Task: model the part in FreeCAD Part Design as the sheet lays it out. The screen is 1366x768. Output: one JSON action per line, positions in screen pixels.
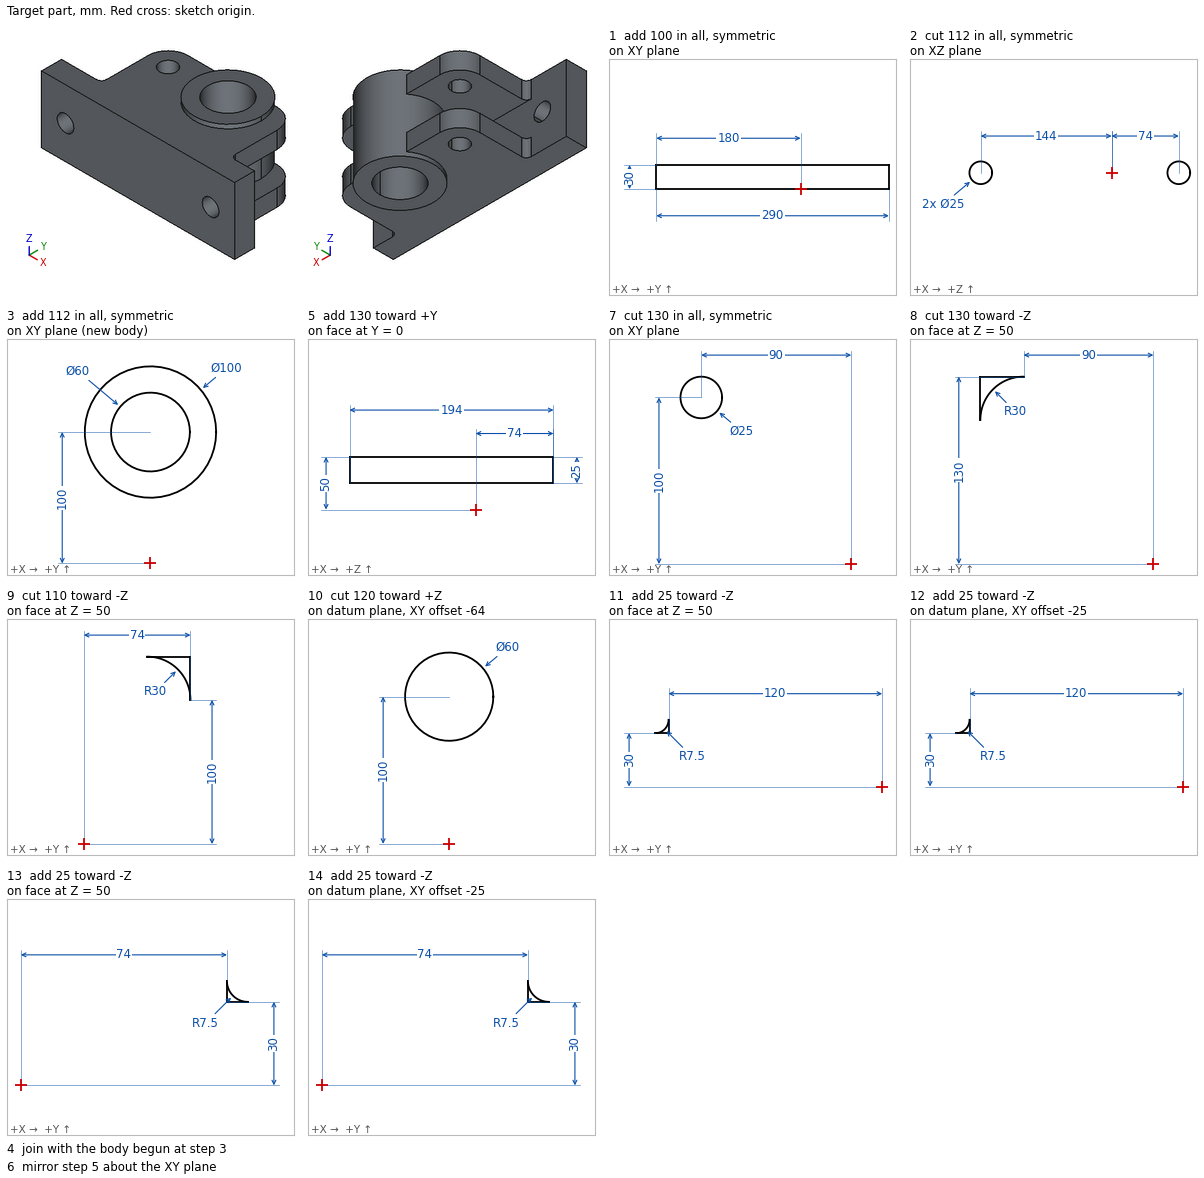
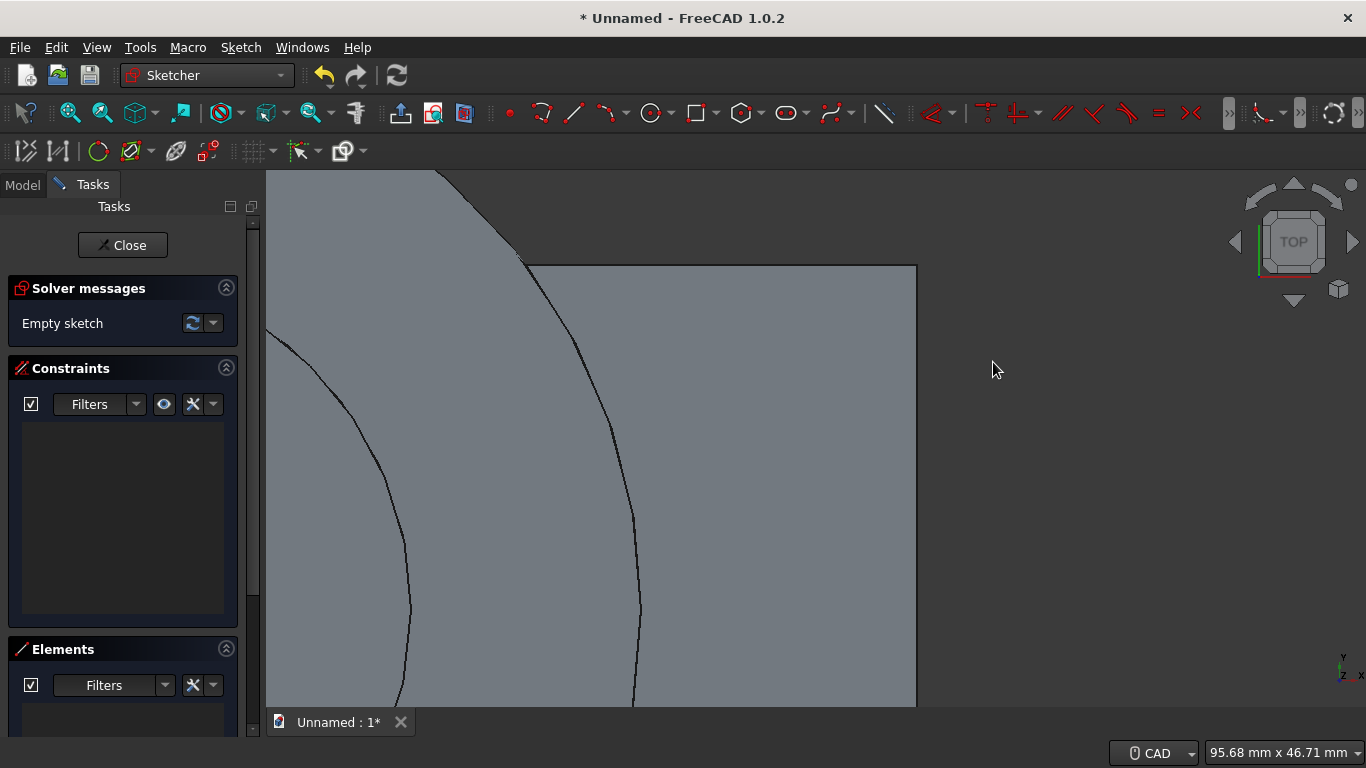
{"action": "left_click", "coordinate": [542, 114]}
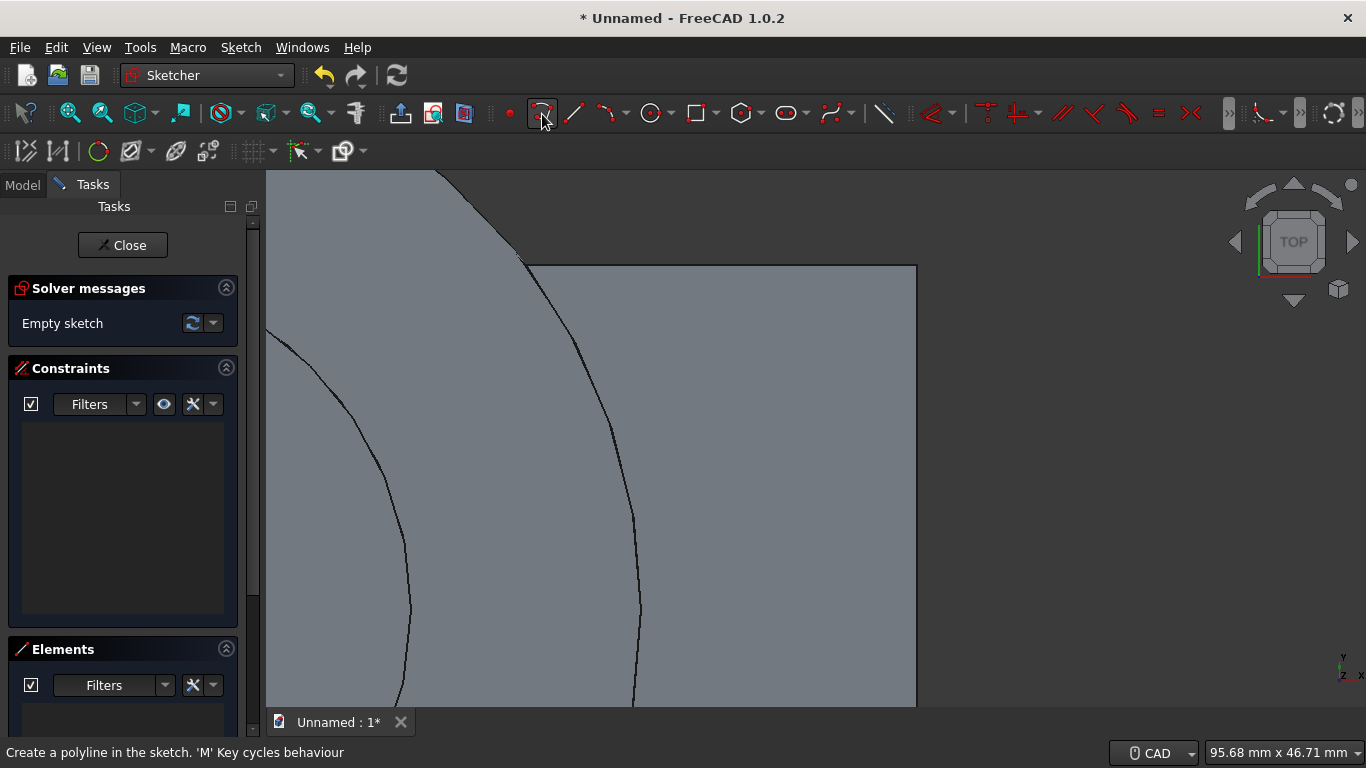
{"action": "left_click", "coordinate": [917, 610]}
{"action": "left_click", "coordinate": [917, 265]}
{"action": "left_click", "coordinate": [572, 265]}
{"action": "right_click", "coordinate": [572, 265]}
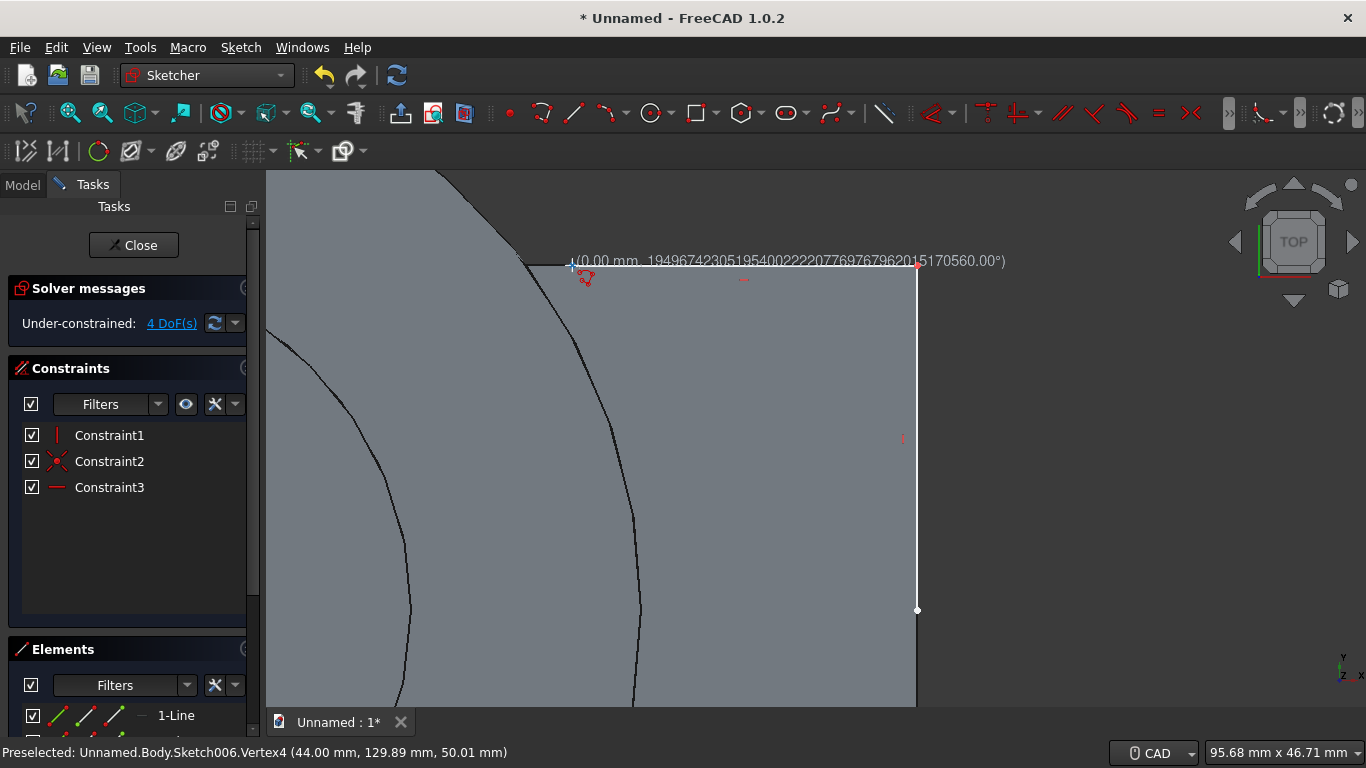
{"action": "left_click", "coordinate": [606, 114]}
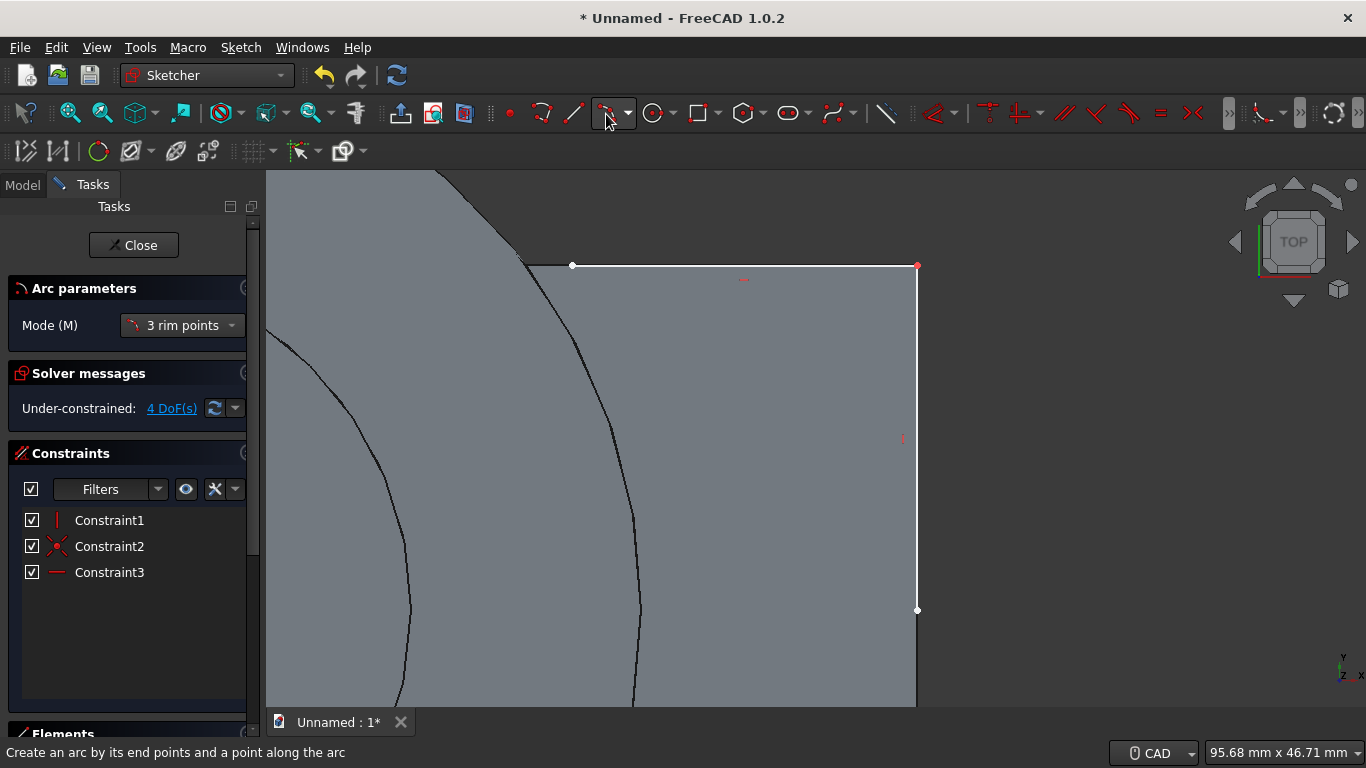
{"action": "left_click", "coordinate": [572, 266]}
{"action": "left_click", "coordinate": [917, 611]}
{"action": "left_click", "coordinate": [816, 366]}
{"action": "key", "text": "Escape"}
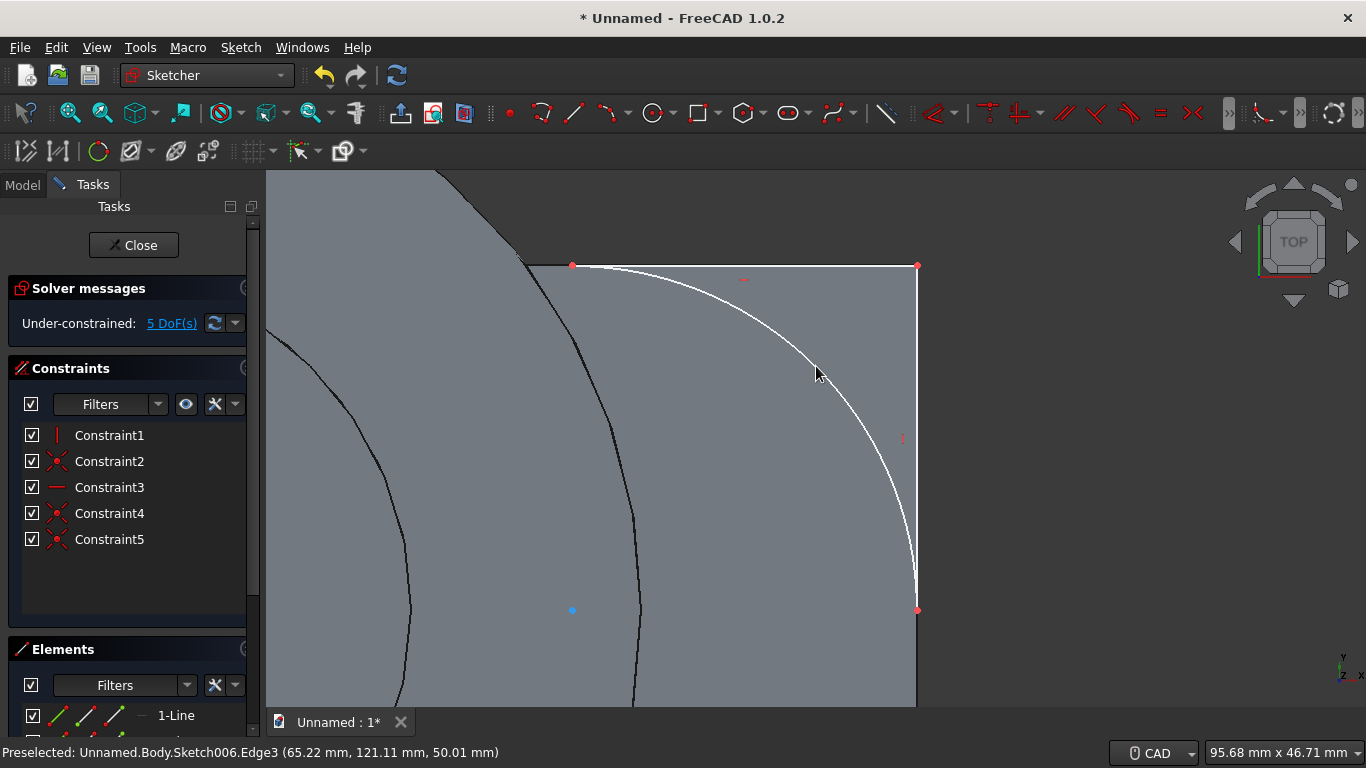
{"action": "left_click", "coordinate": [917, 508]}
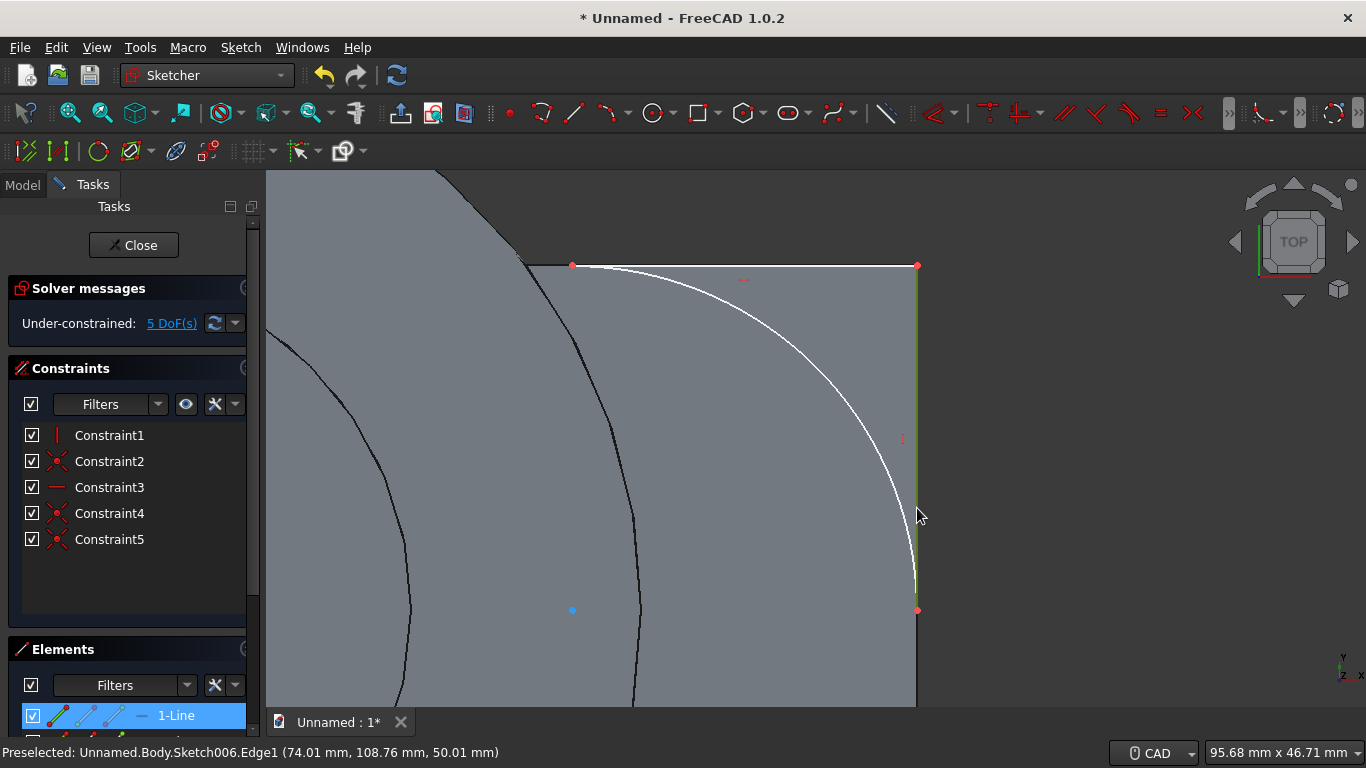
{"action": "left_click", "coordinate": [879, 454]}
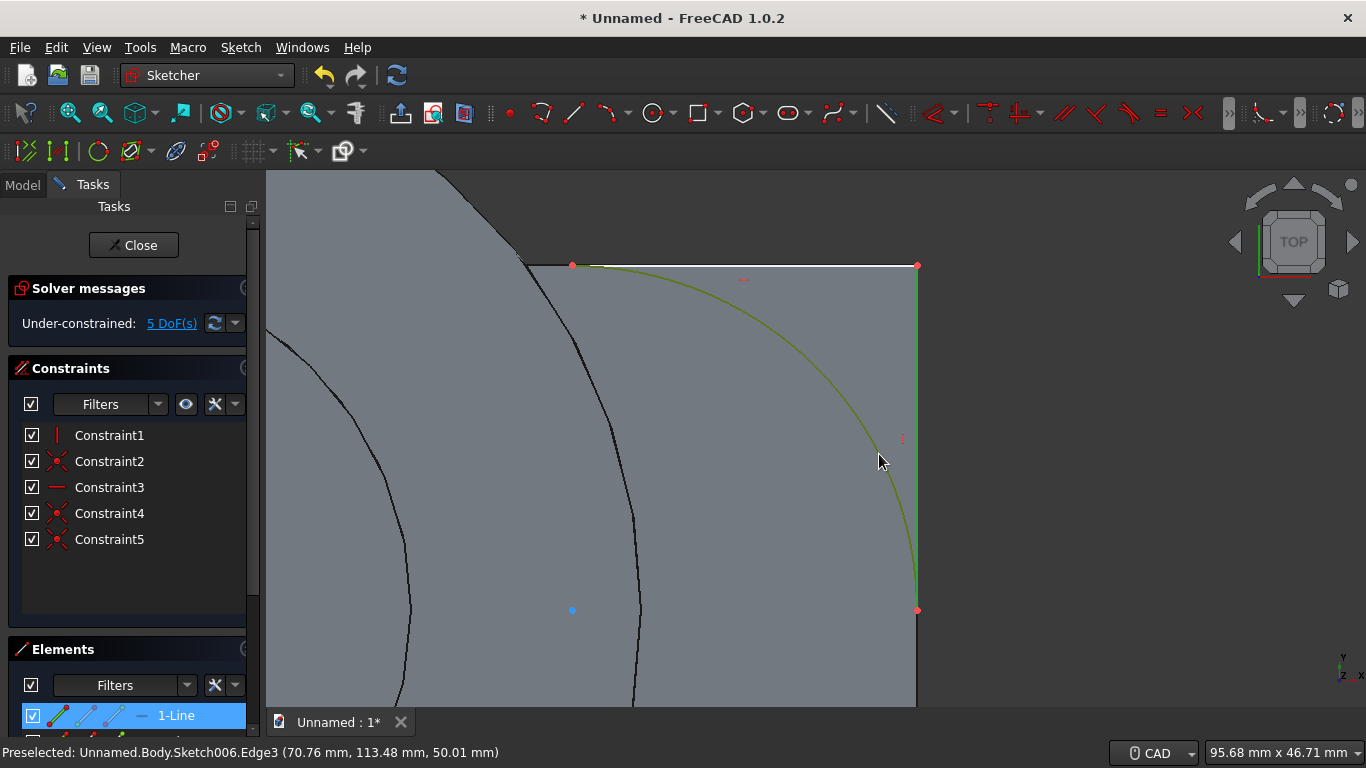
{"action": "left_click", "coordinate": [1130, 114]}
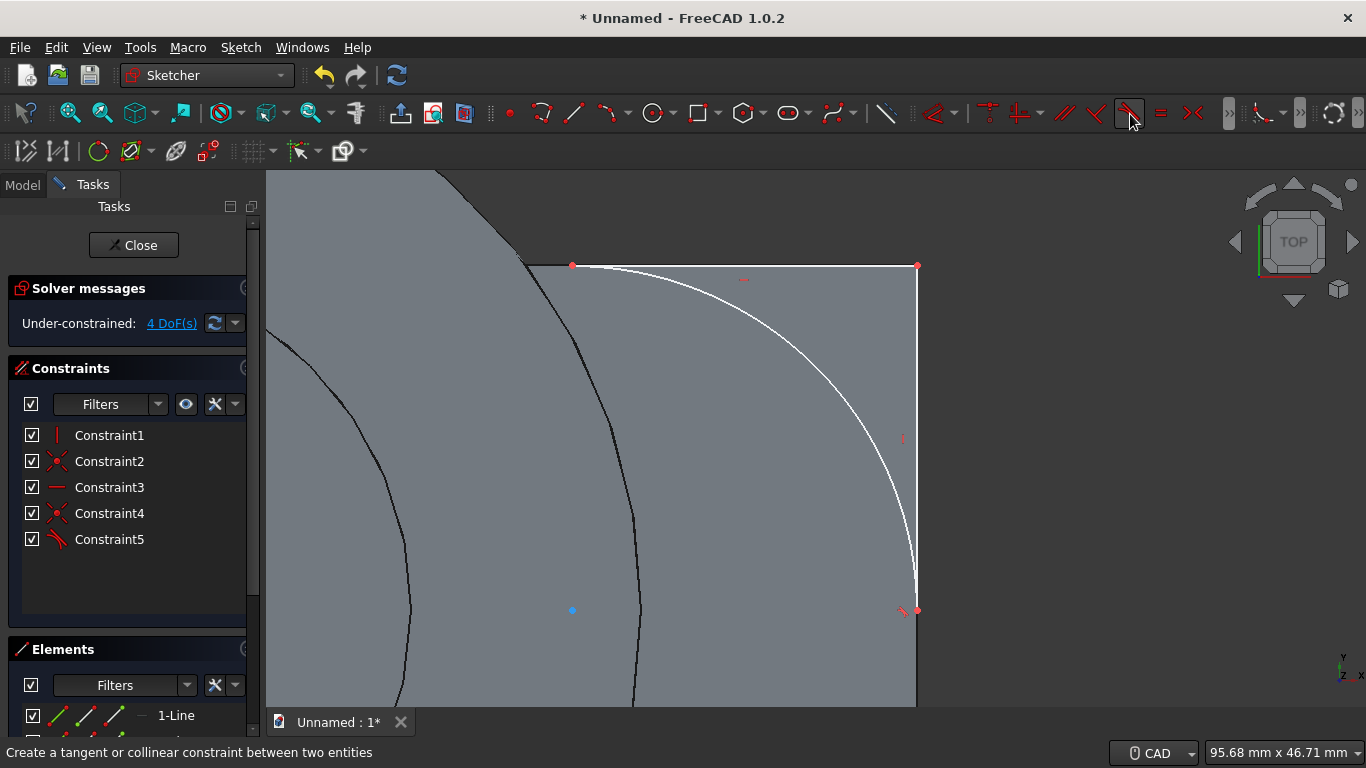
{"action": "left_click", "coordinate": [814, 266]}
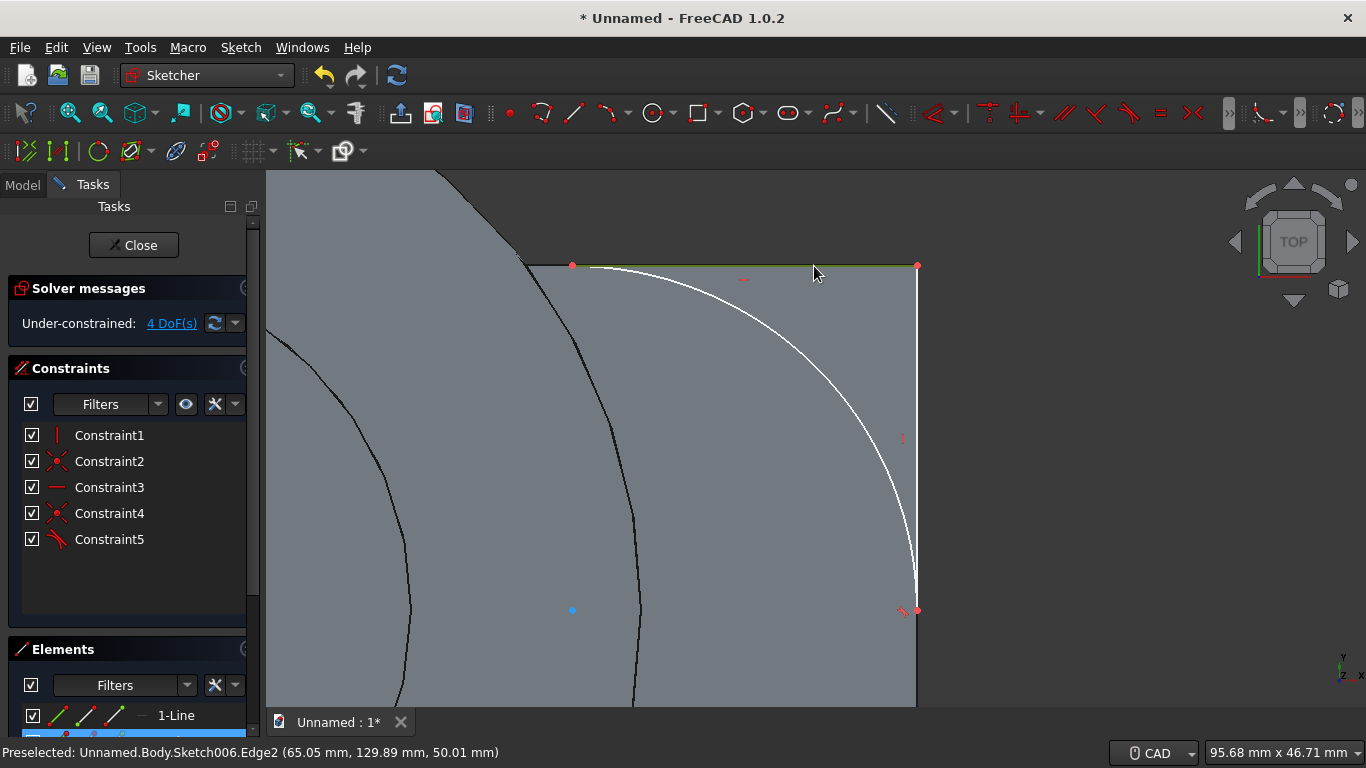
{"action": "left_click", "coordinate": [879, 454]}